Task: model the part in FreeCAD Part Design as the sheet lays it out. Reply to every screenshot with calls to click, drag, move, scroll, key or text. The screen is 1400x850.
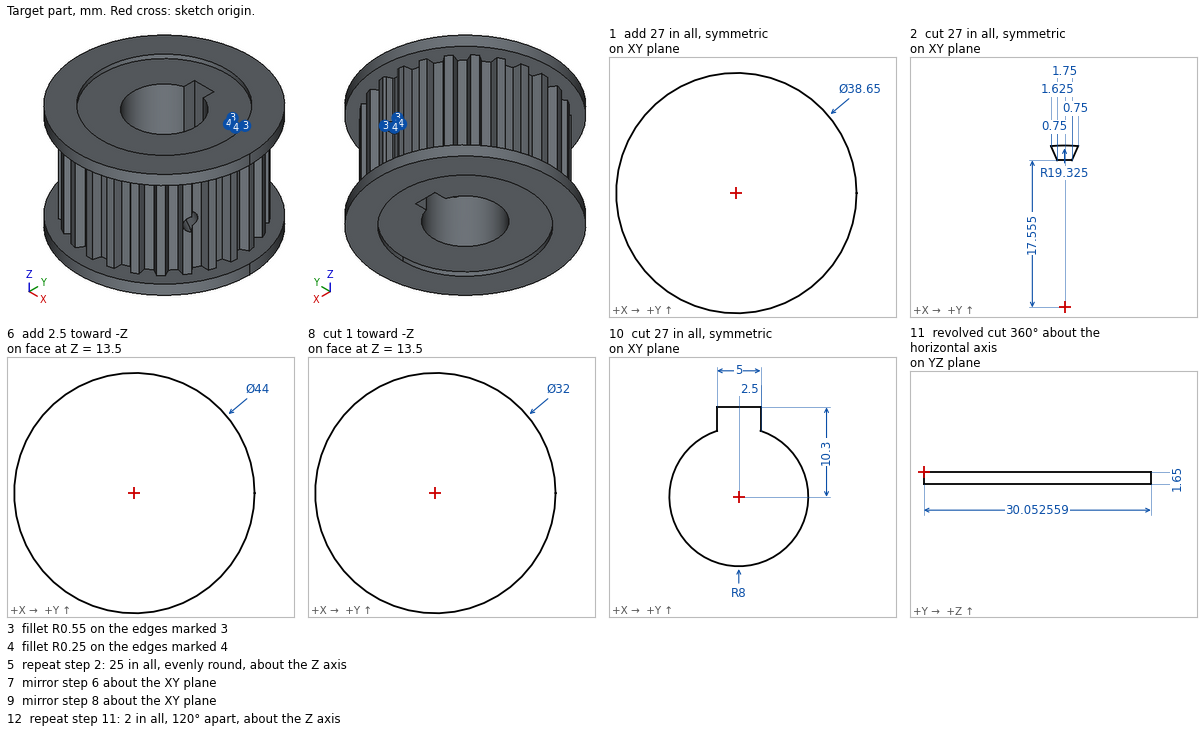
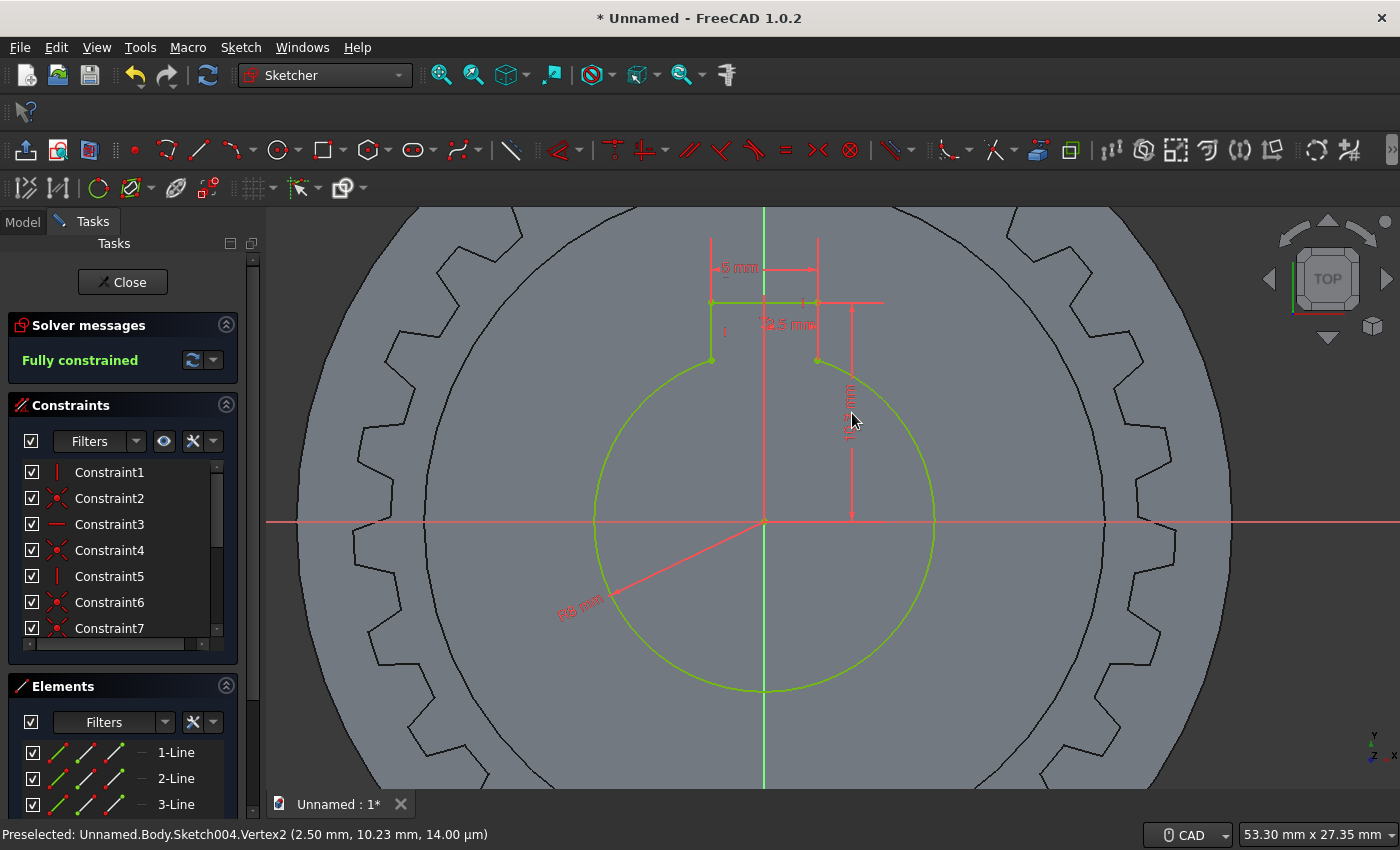
click(123, 282)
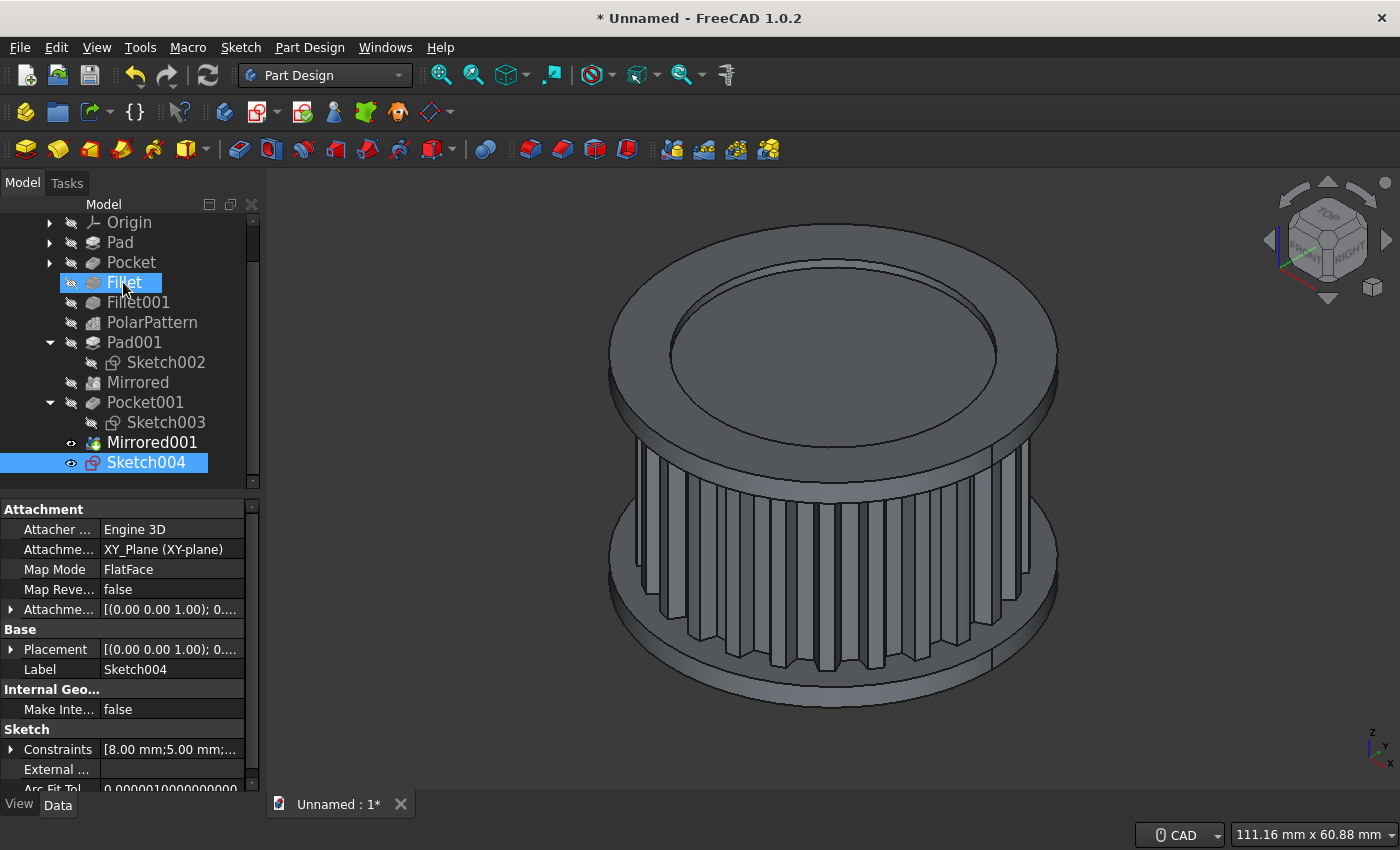
click(240, 150)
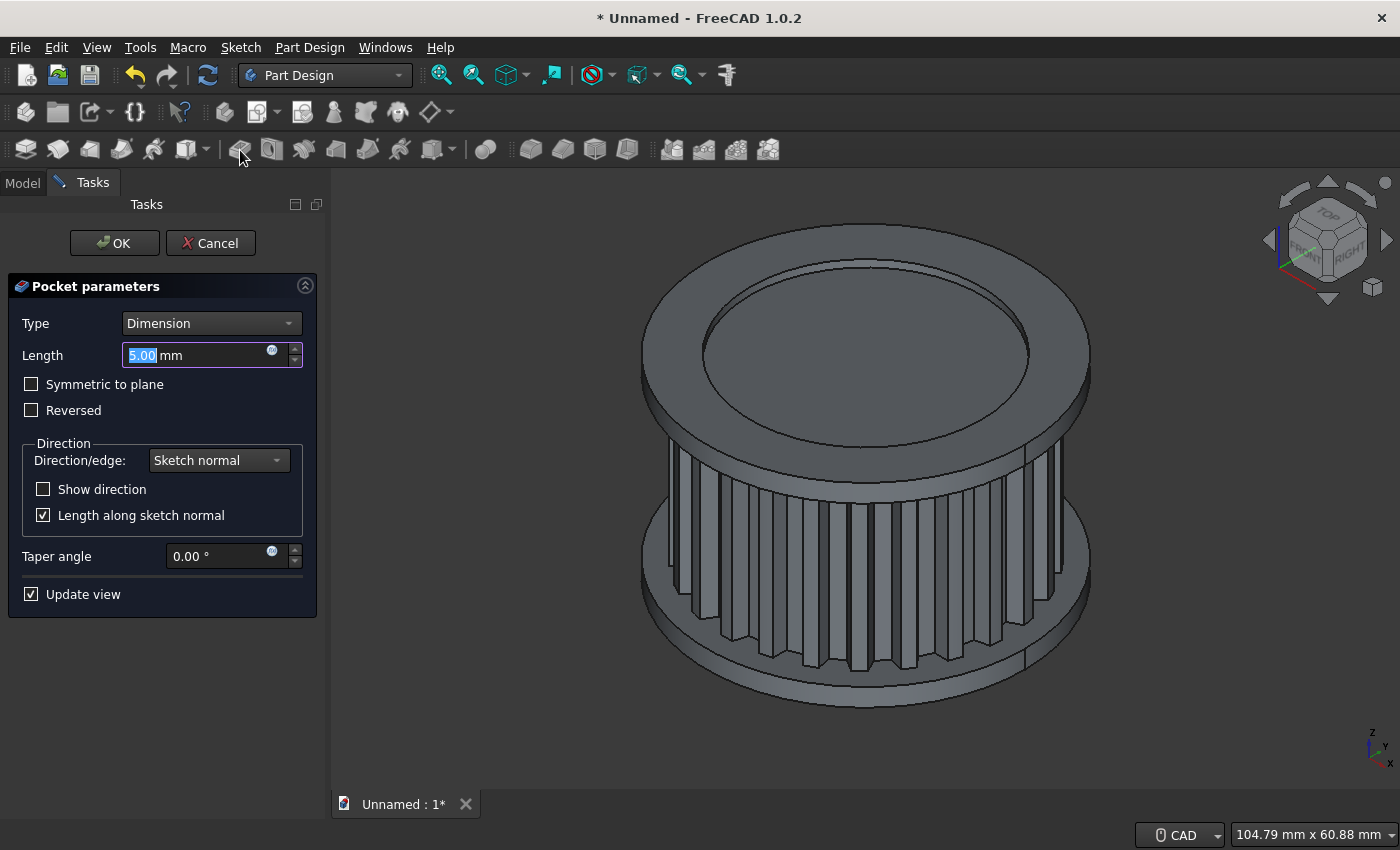
text(27)
key(Tab)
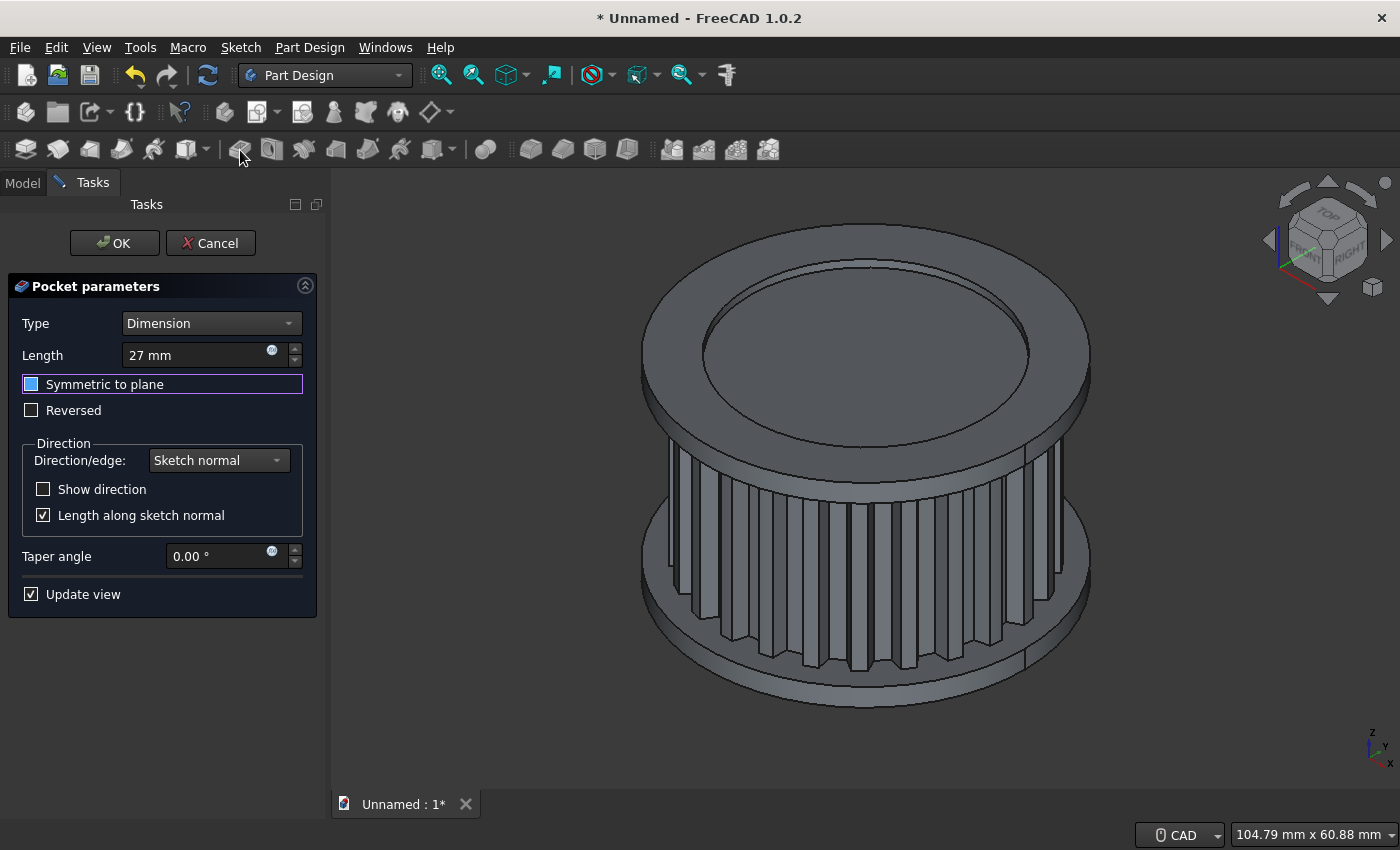
click(30, 384)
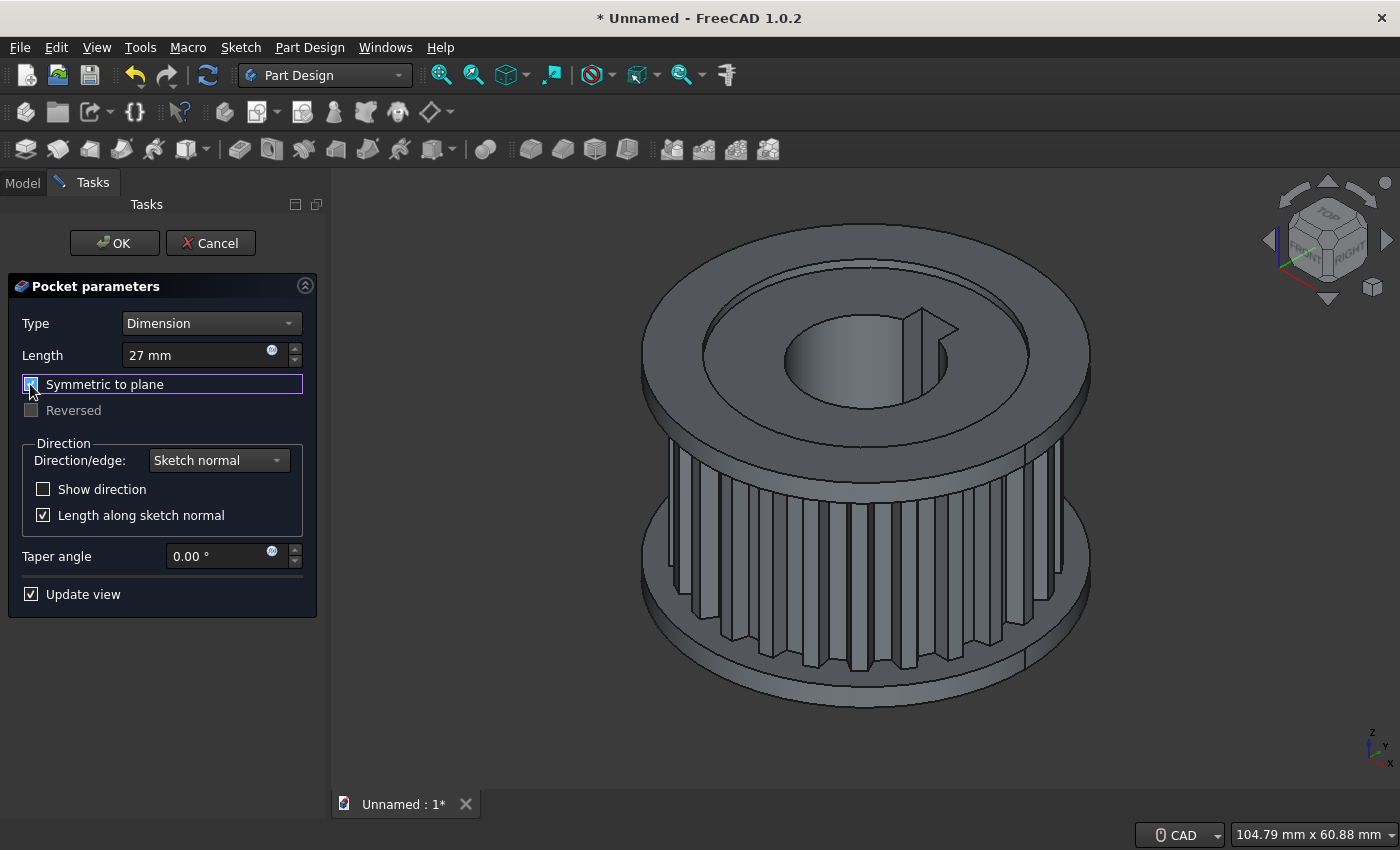
click(115, 243)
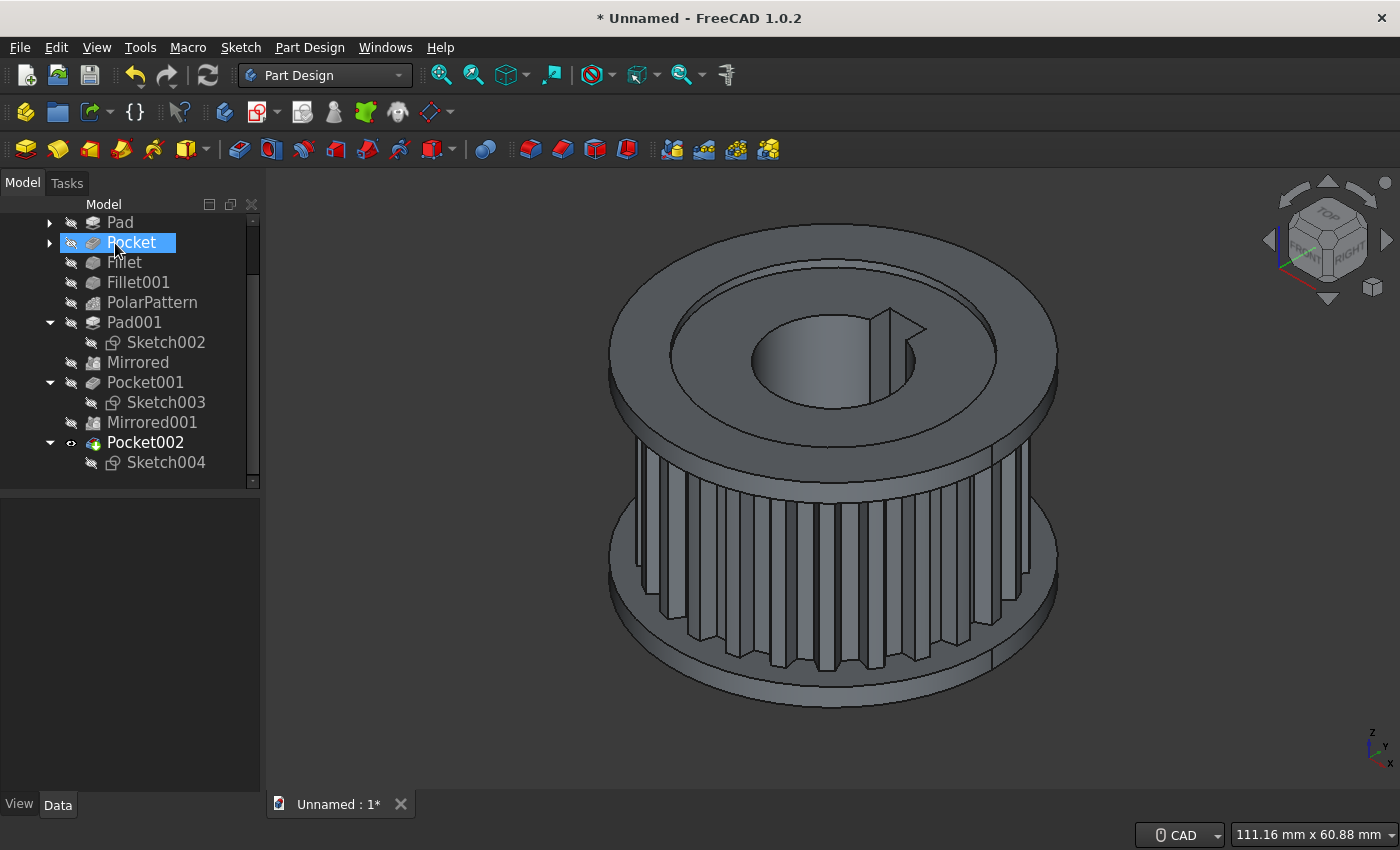
click(258, 112)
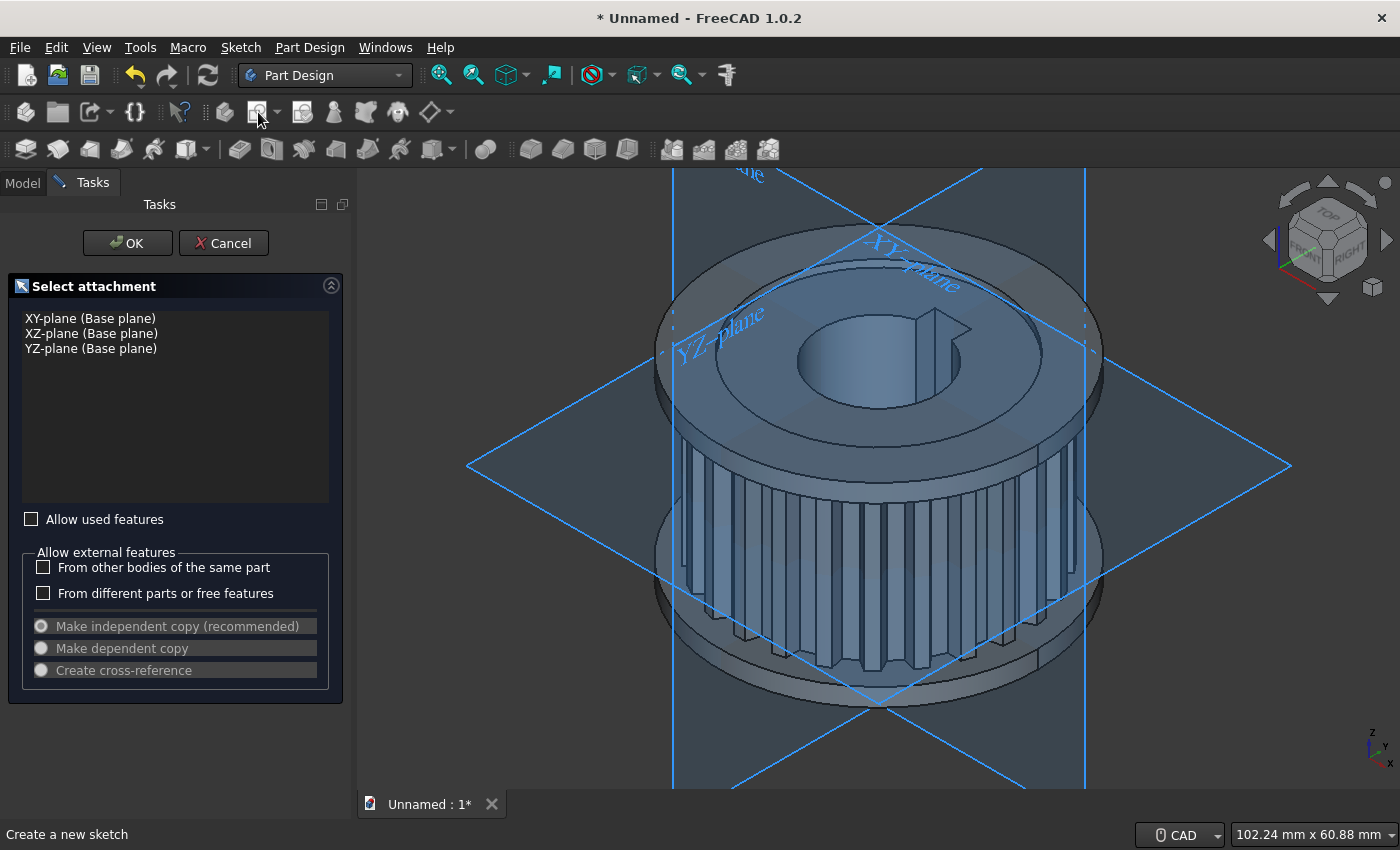
click(82, 348)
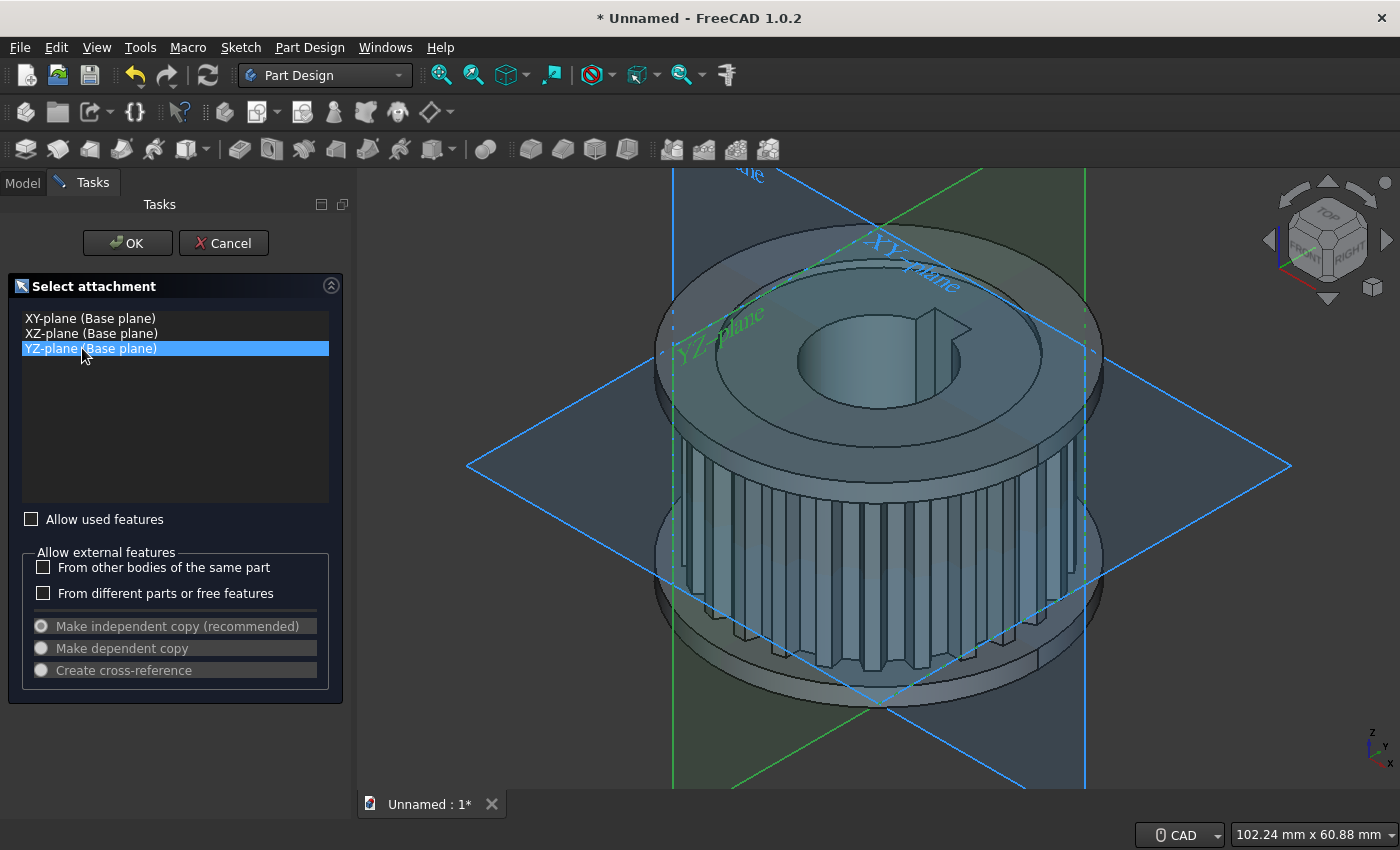
click(128, 243)